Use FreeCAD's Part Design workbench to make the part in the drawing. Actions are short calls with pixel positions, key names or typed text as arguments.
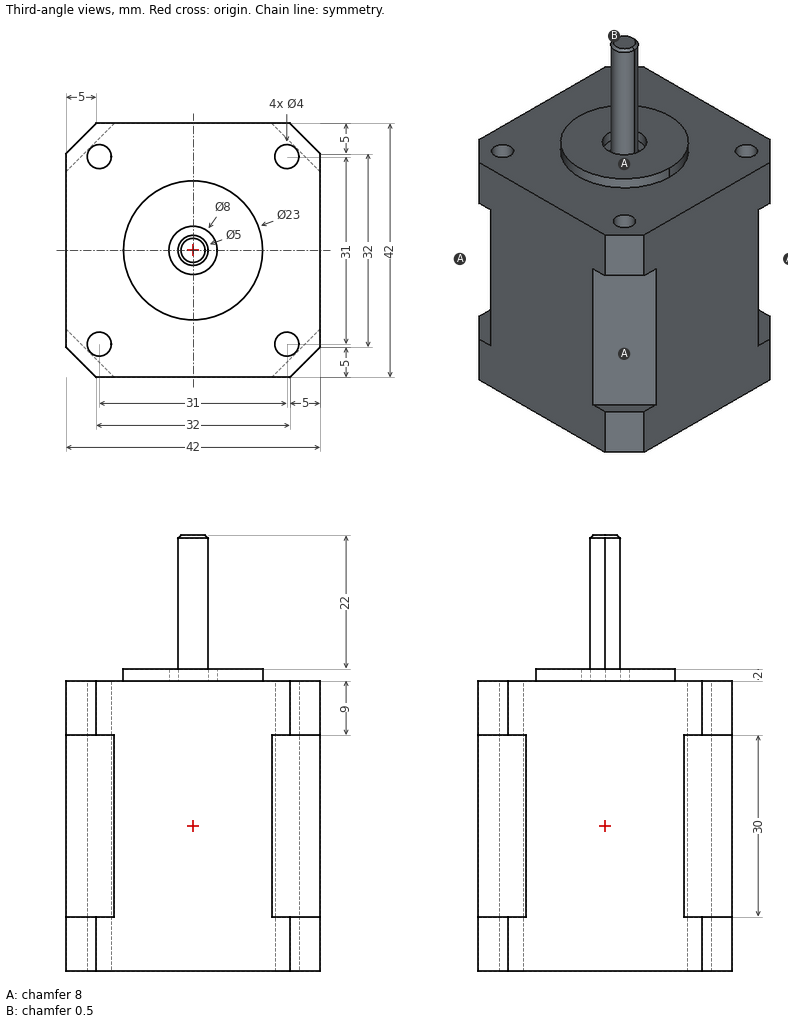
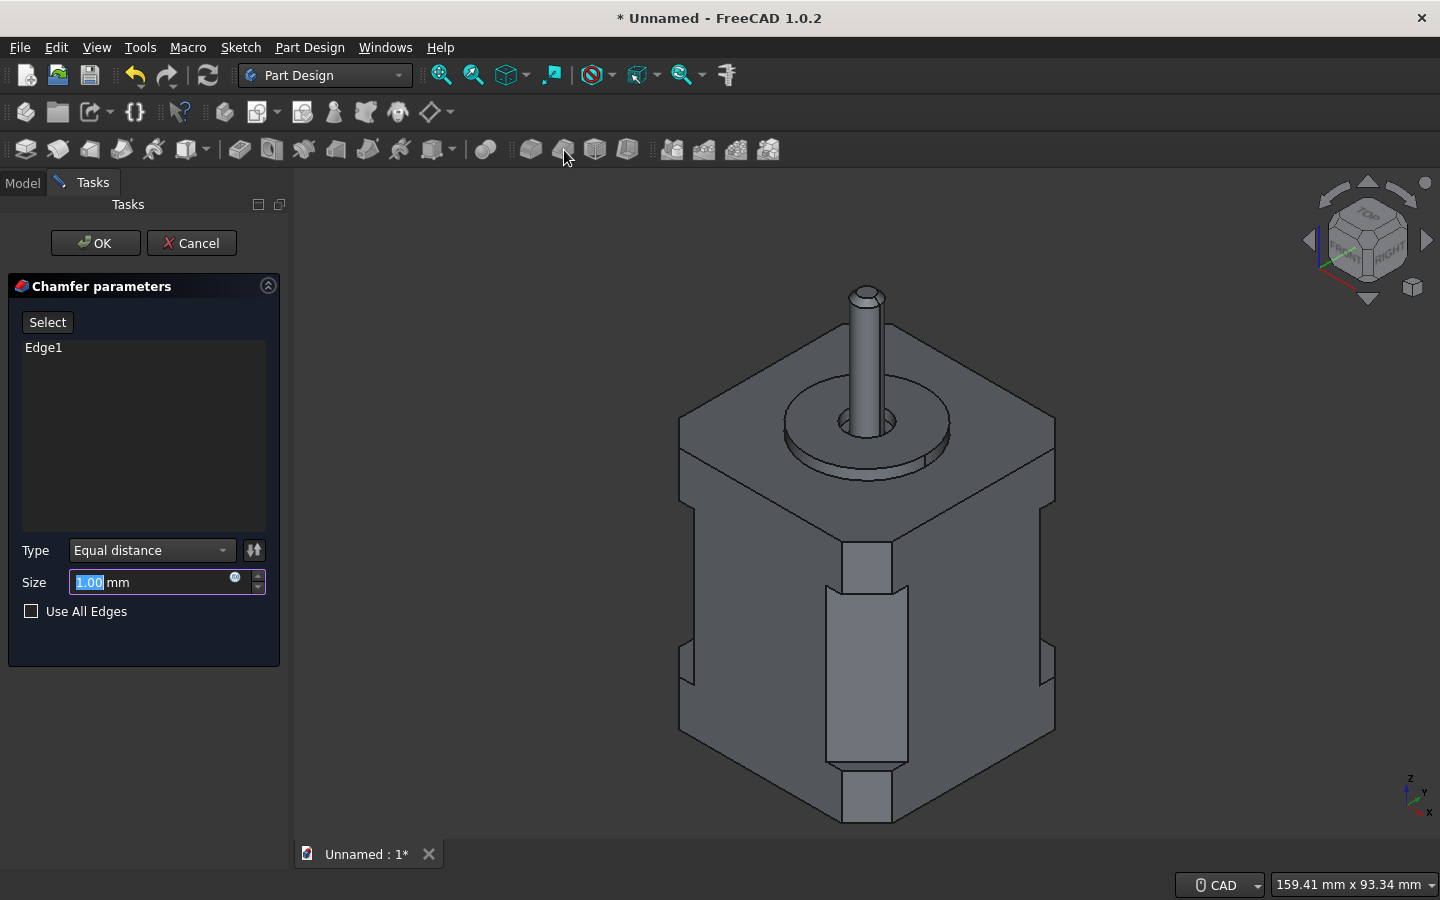
text(0.5)
key(Tab)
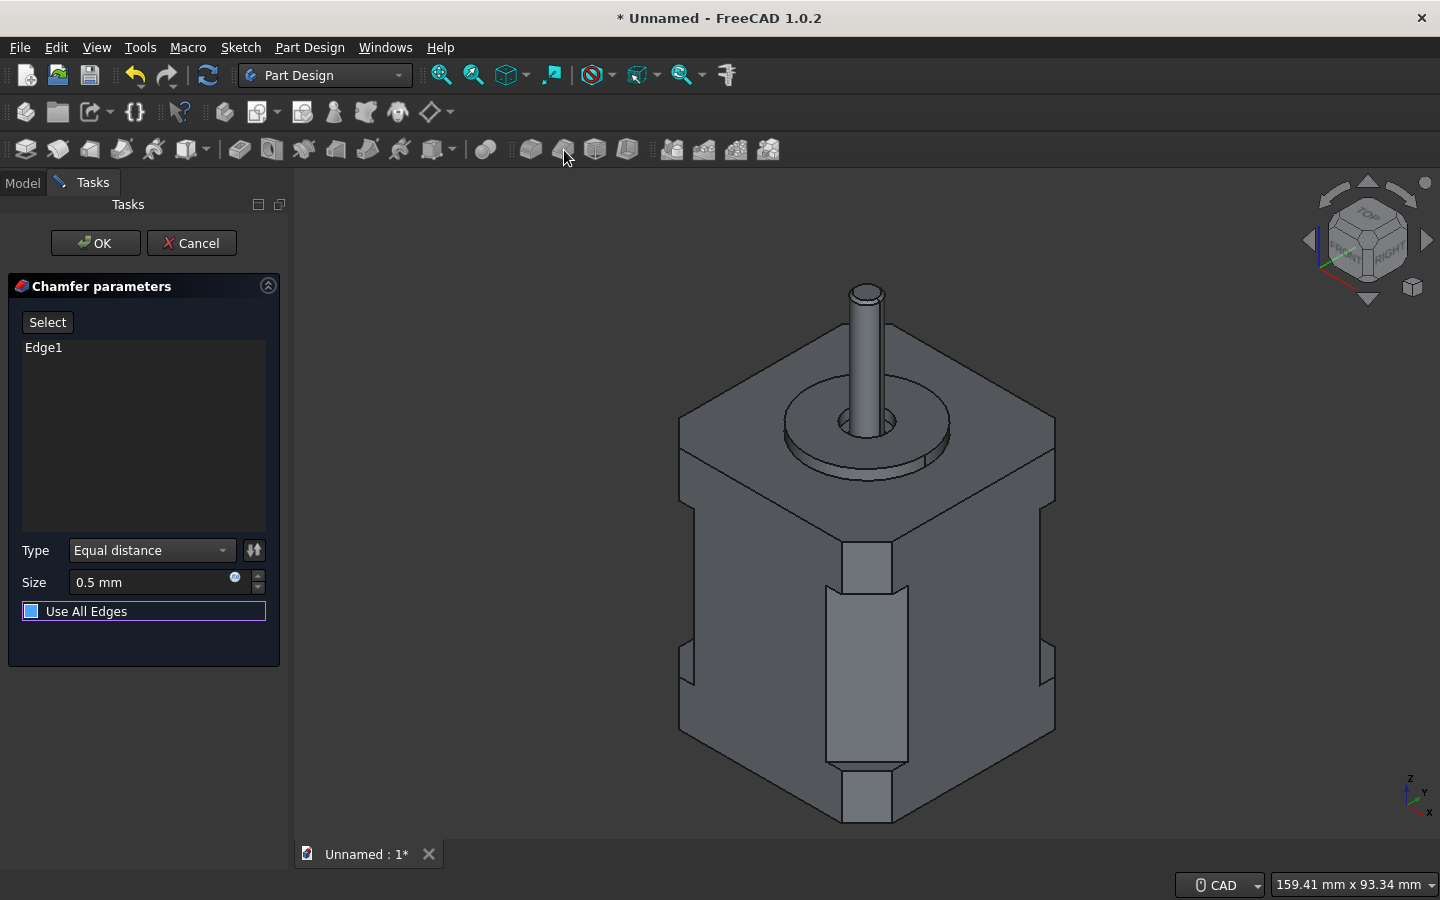
click(96, 243)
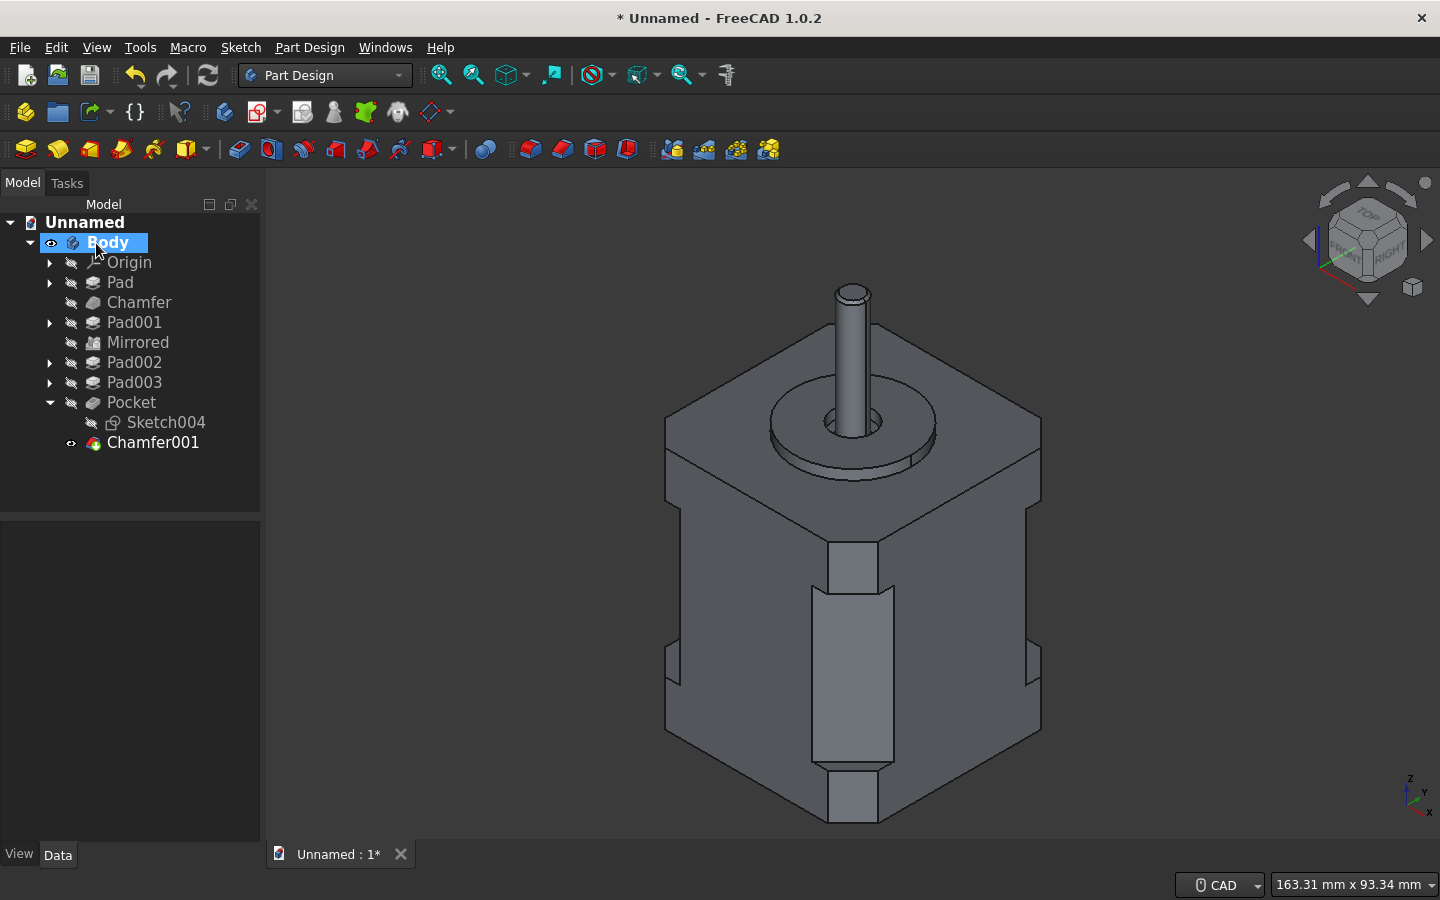
click(975, 432)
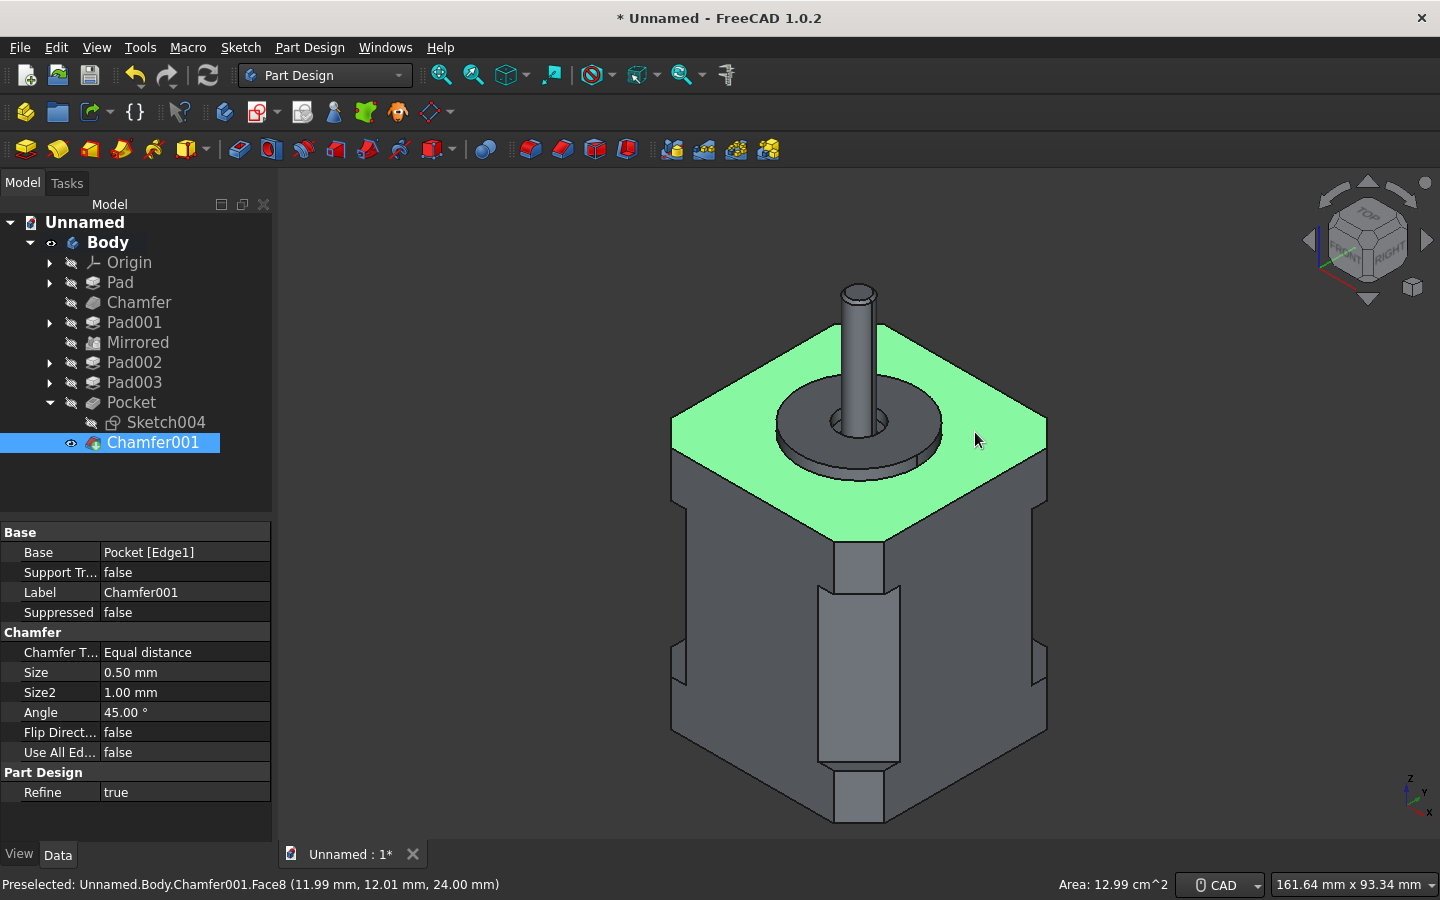
click(258, 112)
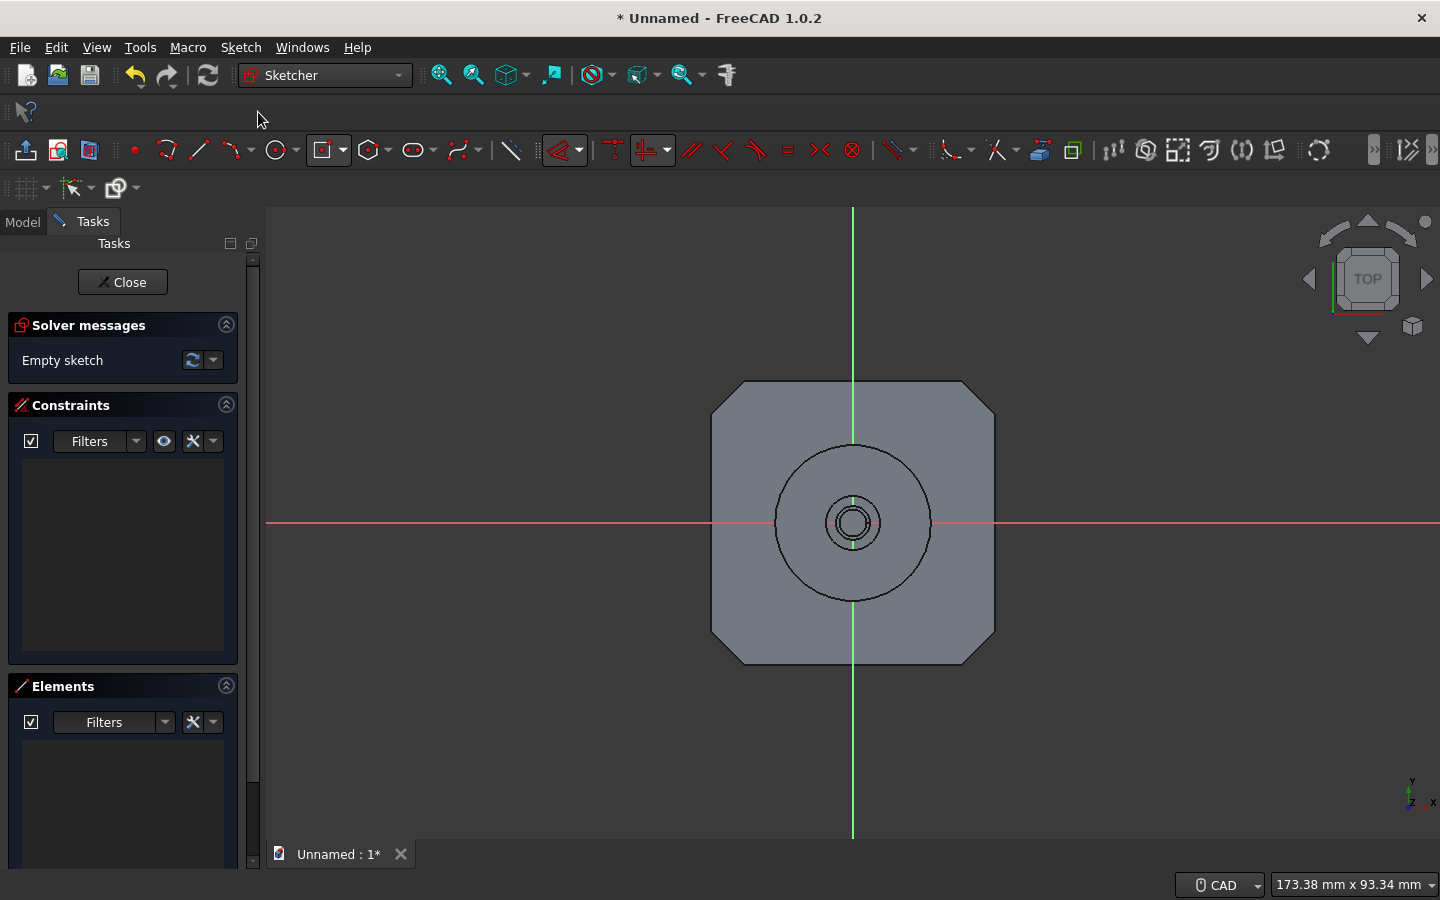
scroll(936, 523, up, 3)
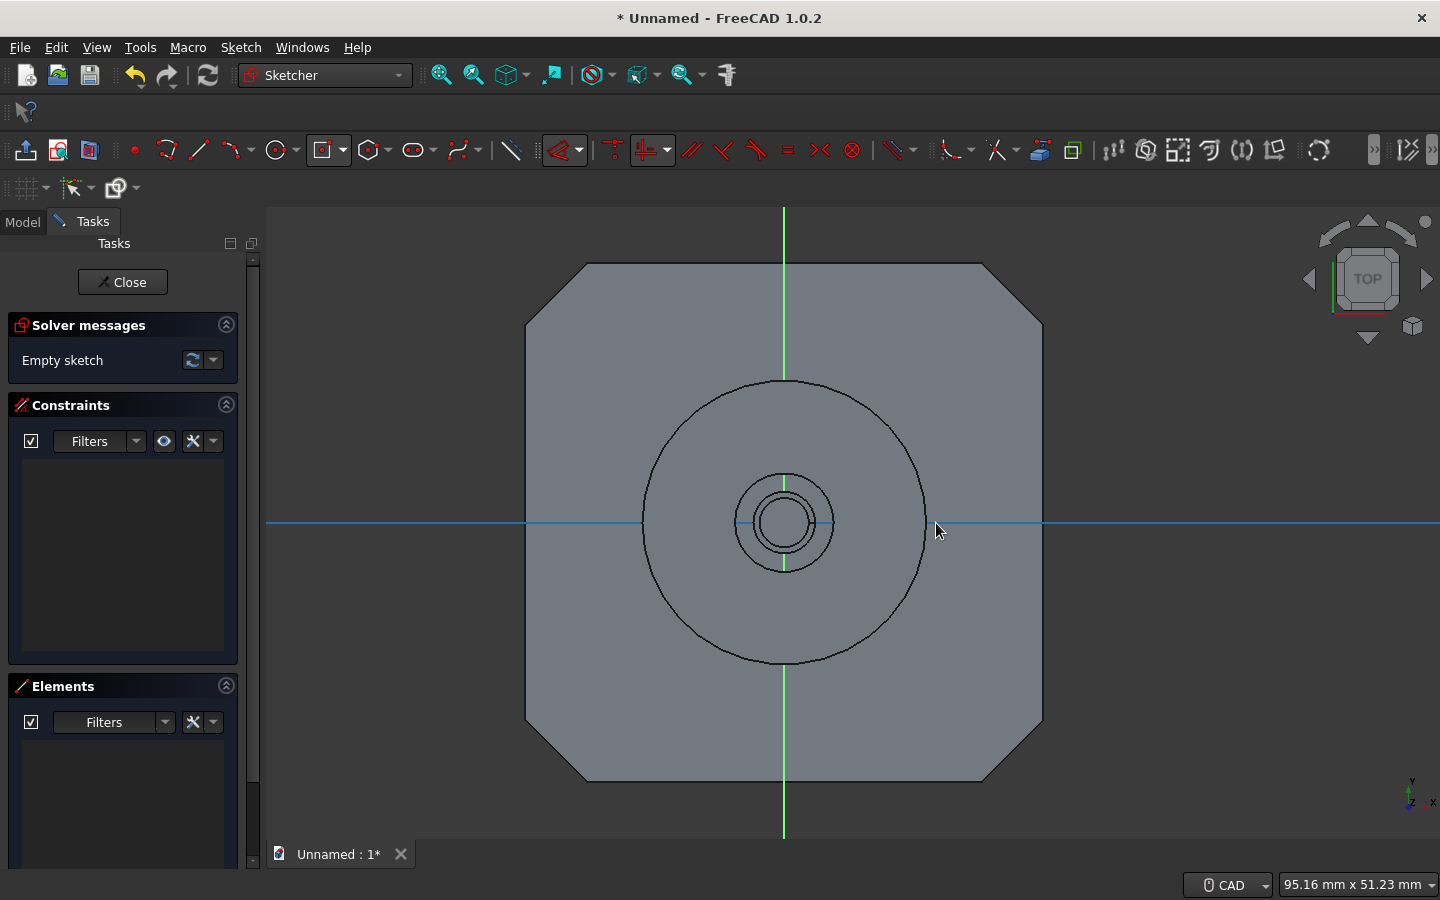
key(g)
key(c)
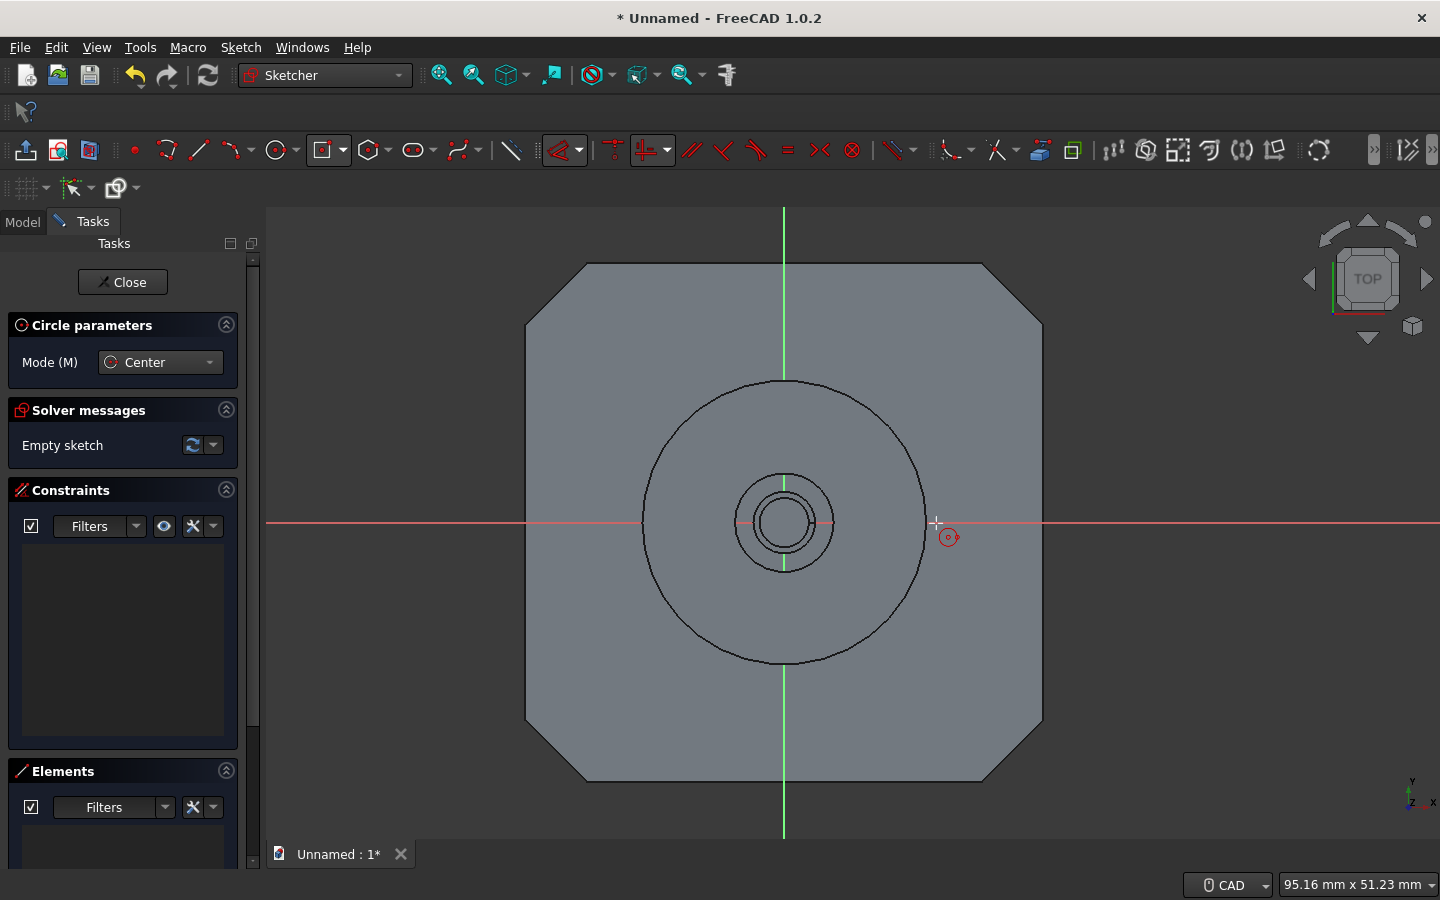
click(976, 331)
move(993, 314)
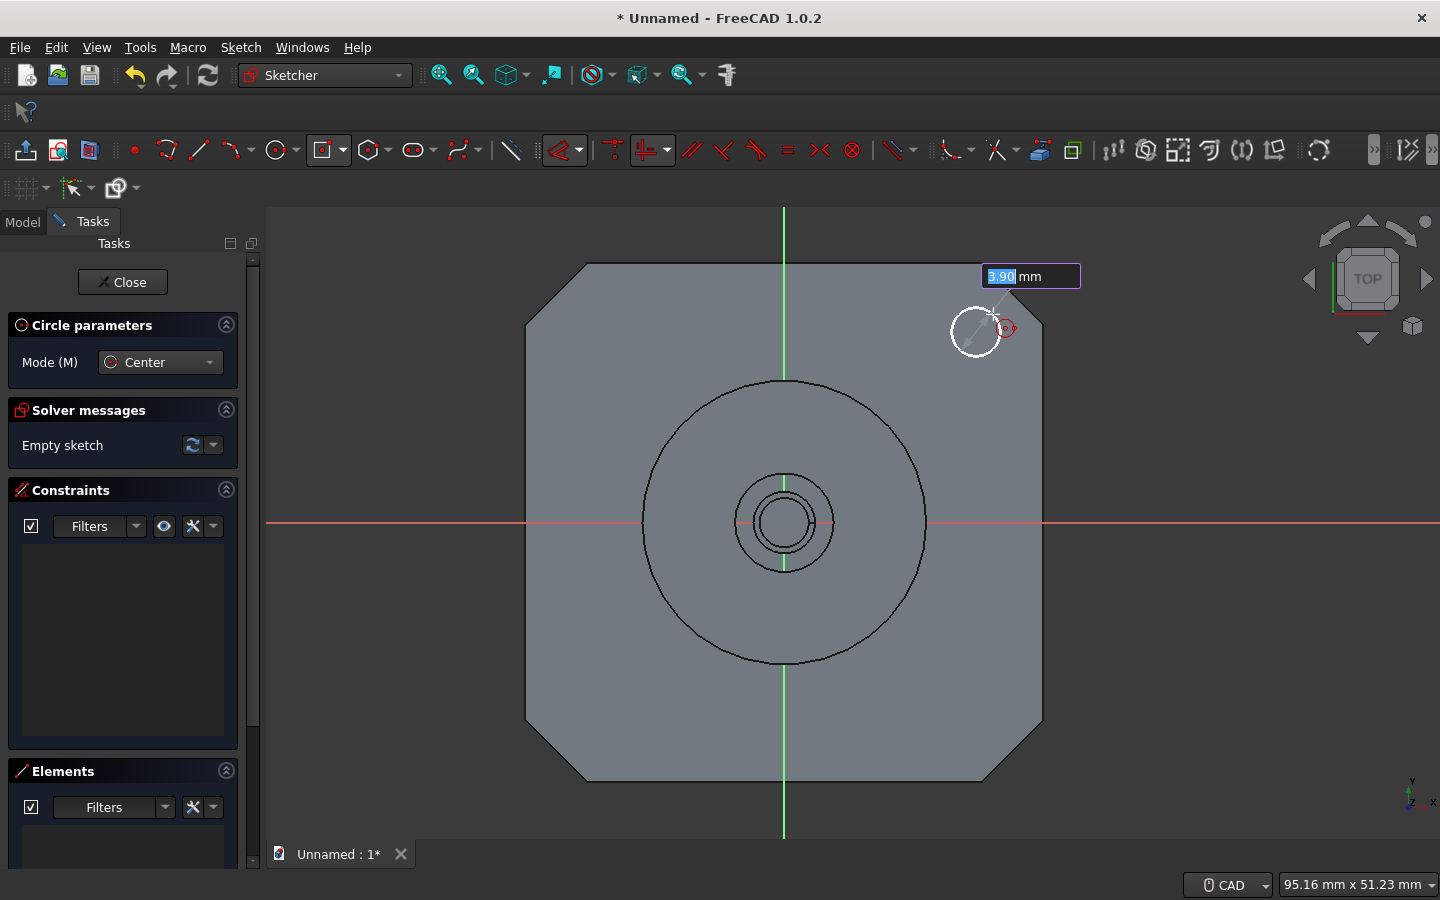
text(4)
key(Return)